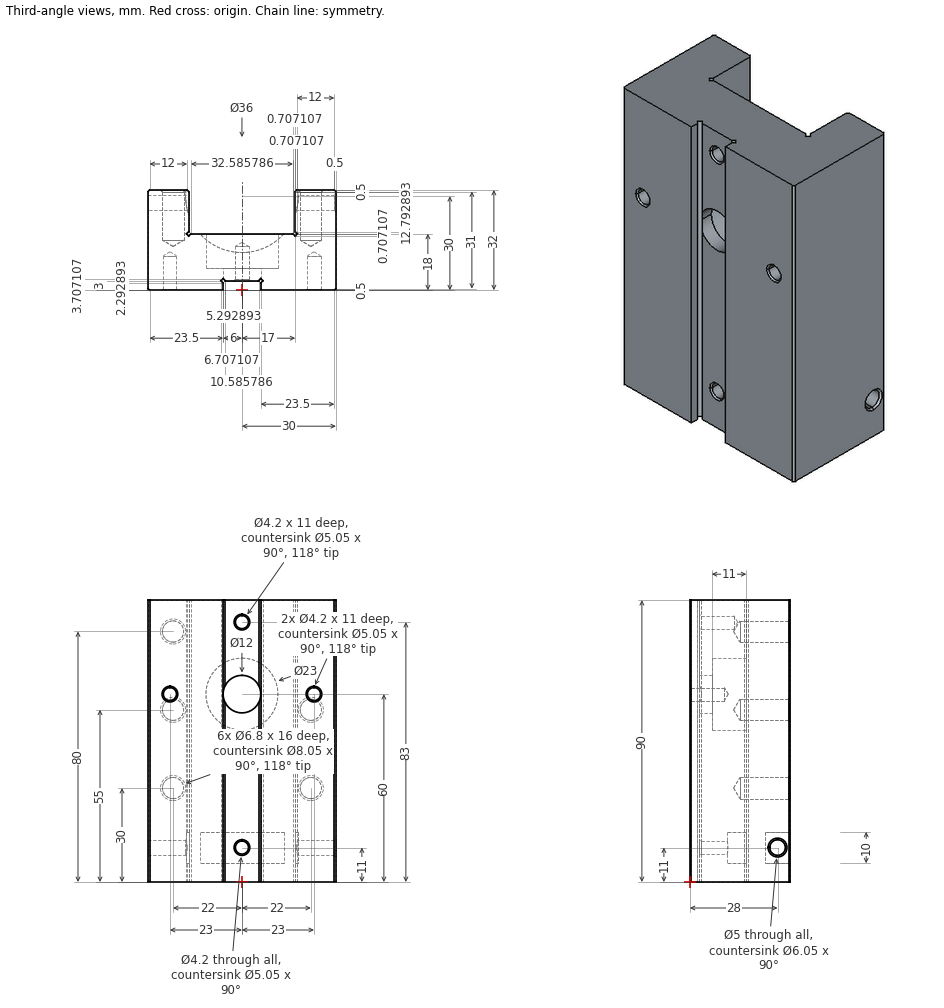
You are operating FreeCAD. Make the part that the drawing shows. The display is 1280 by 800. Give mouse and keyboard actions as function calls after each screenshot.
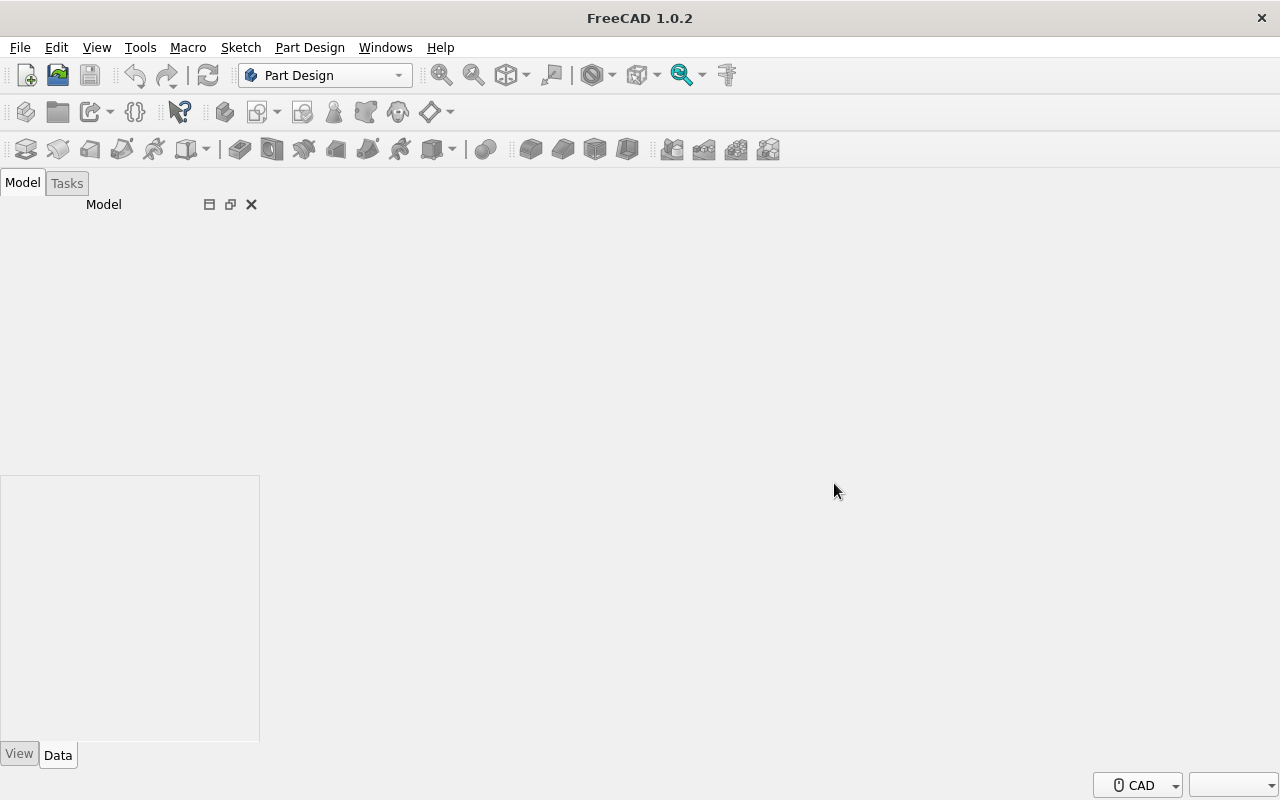
click(26, 76)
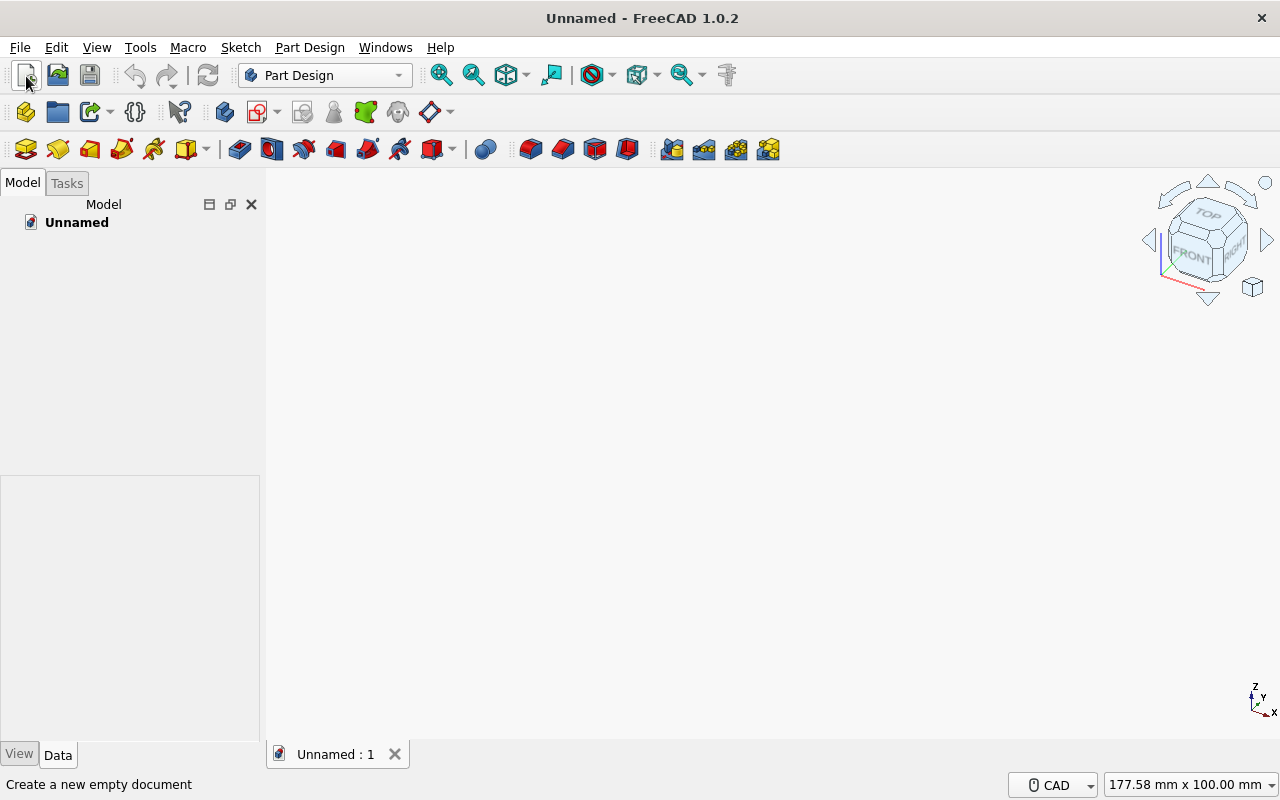
click(258, 112)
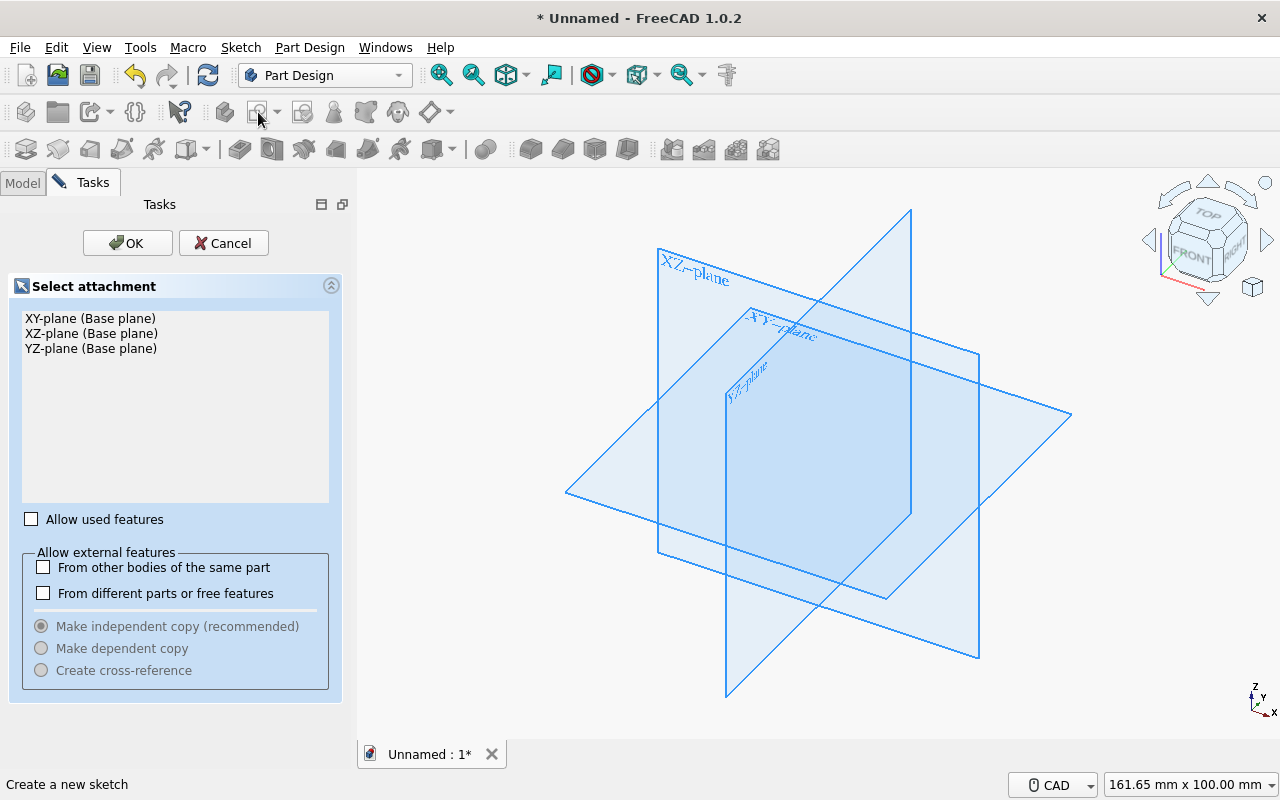
click(82, 318)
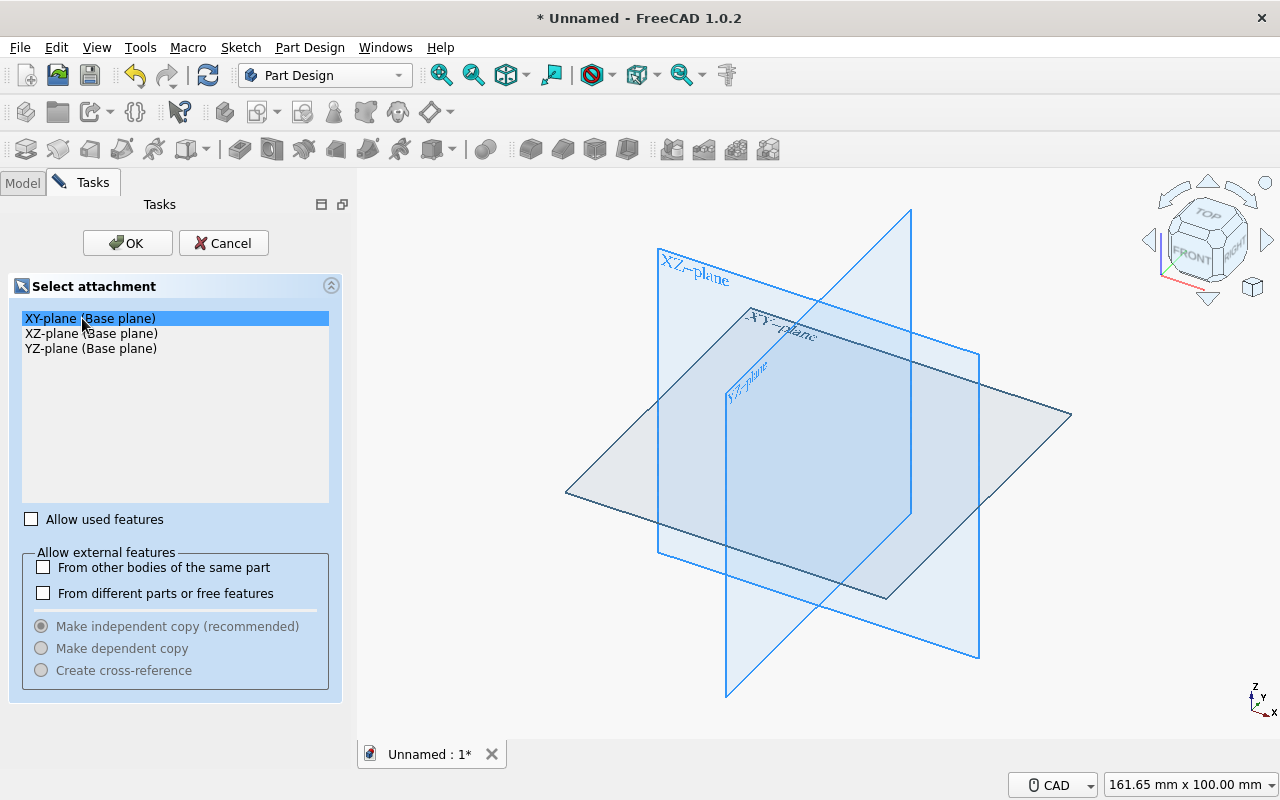
click(128, 243)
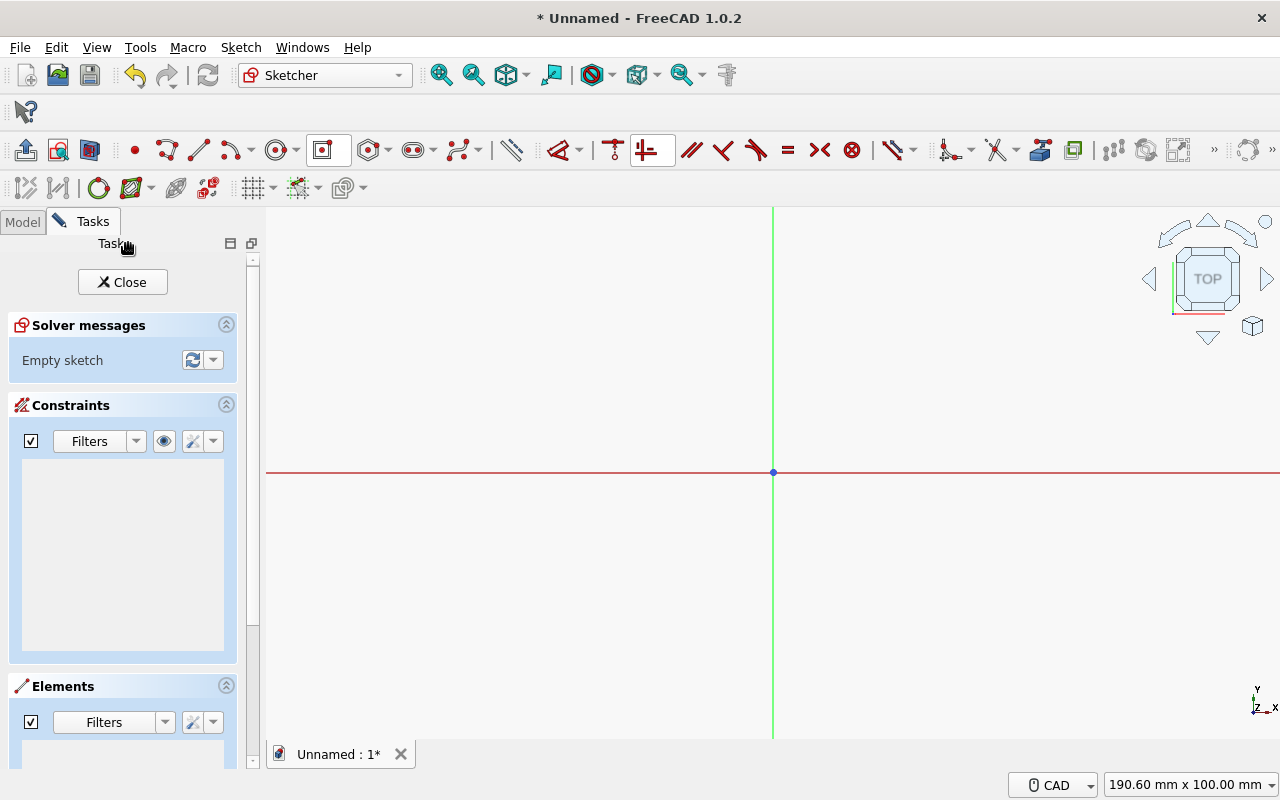
scroll(856, 284, up, 3)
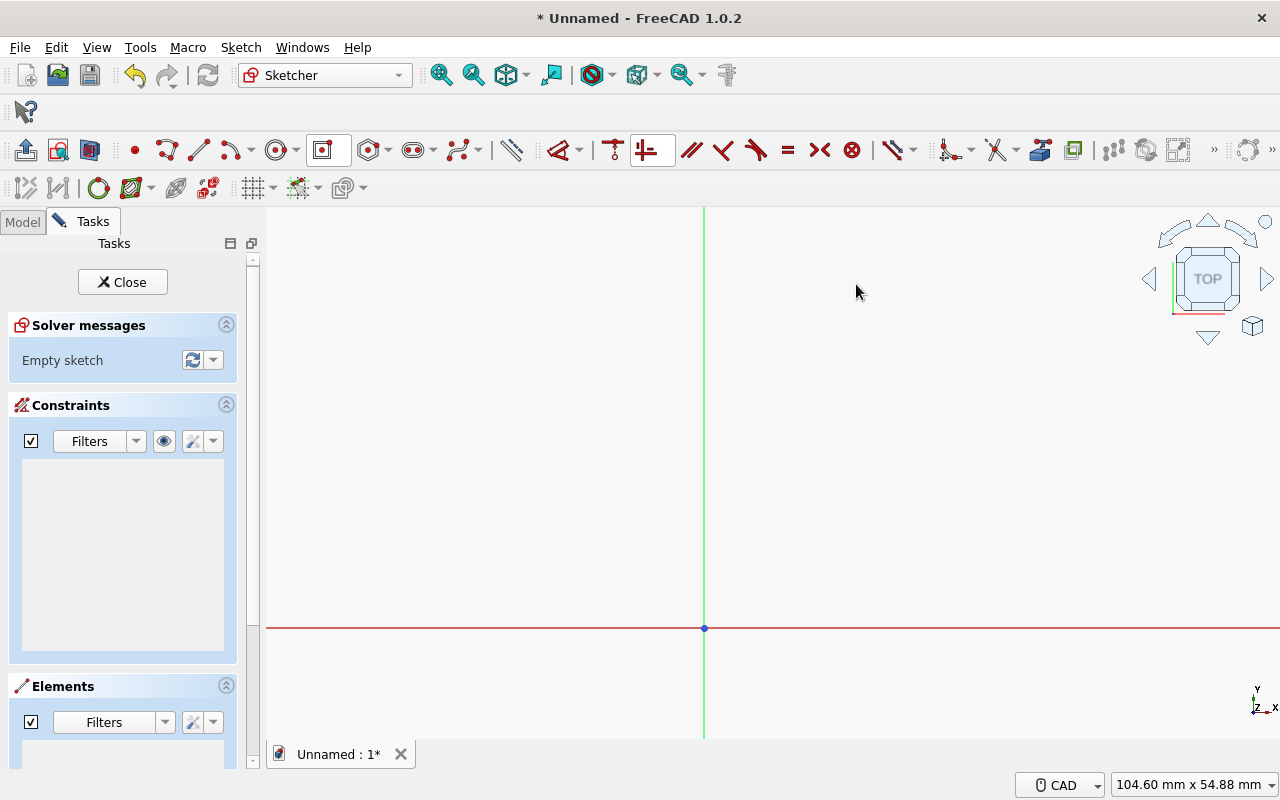
click(168, 150)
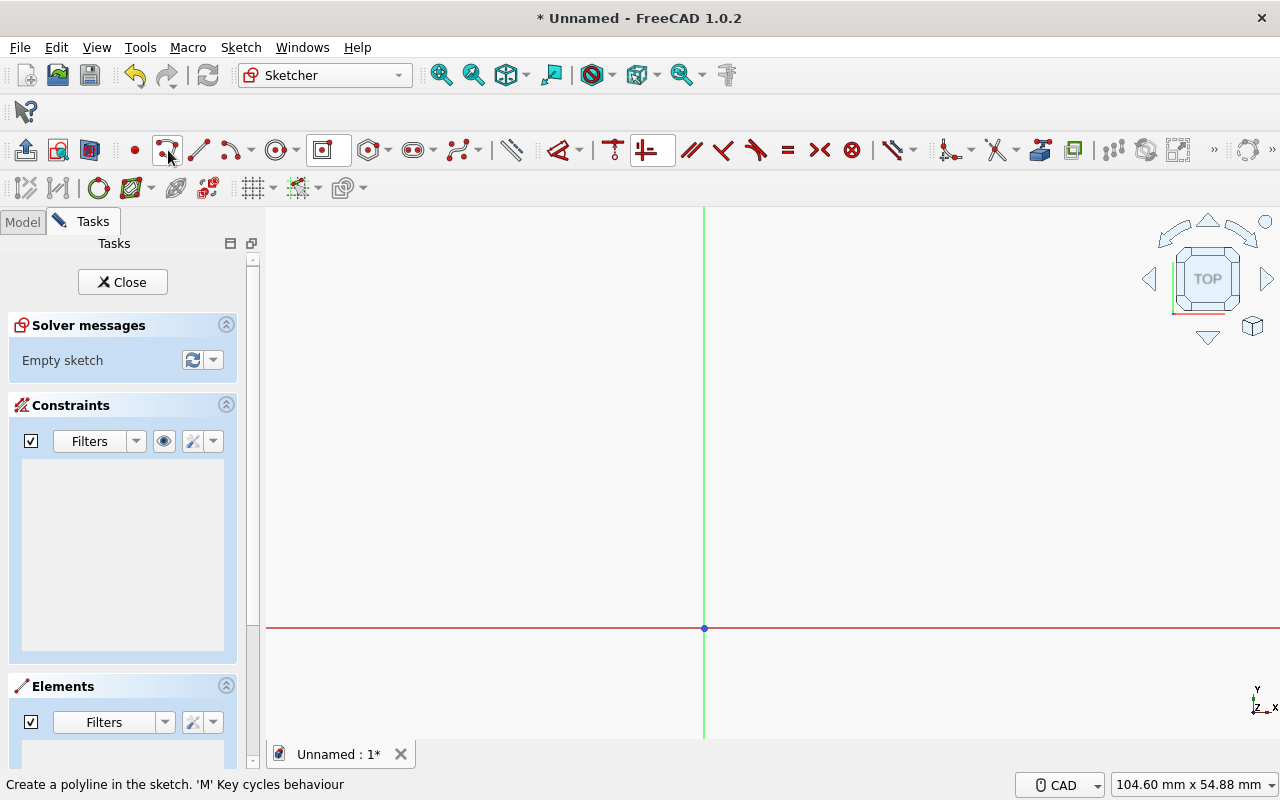
click(646, 628)
click(646, 606)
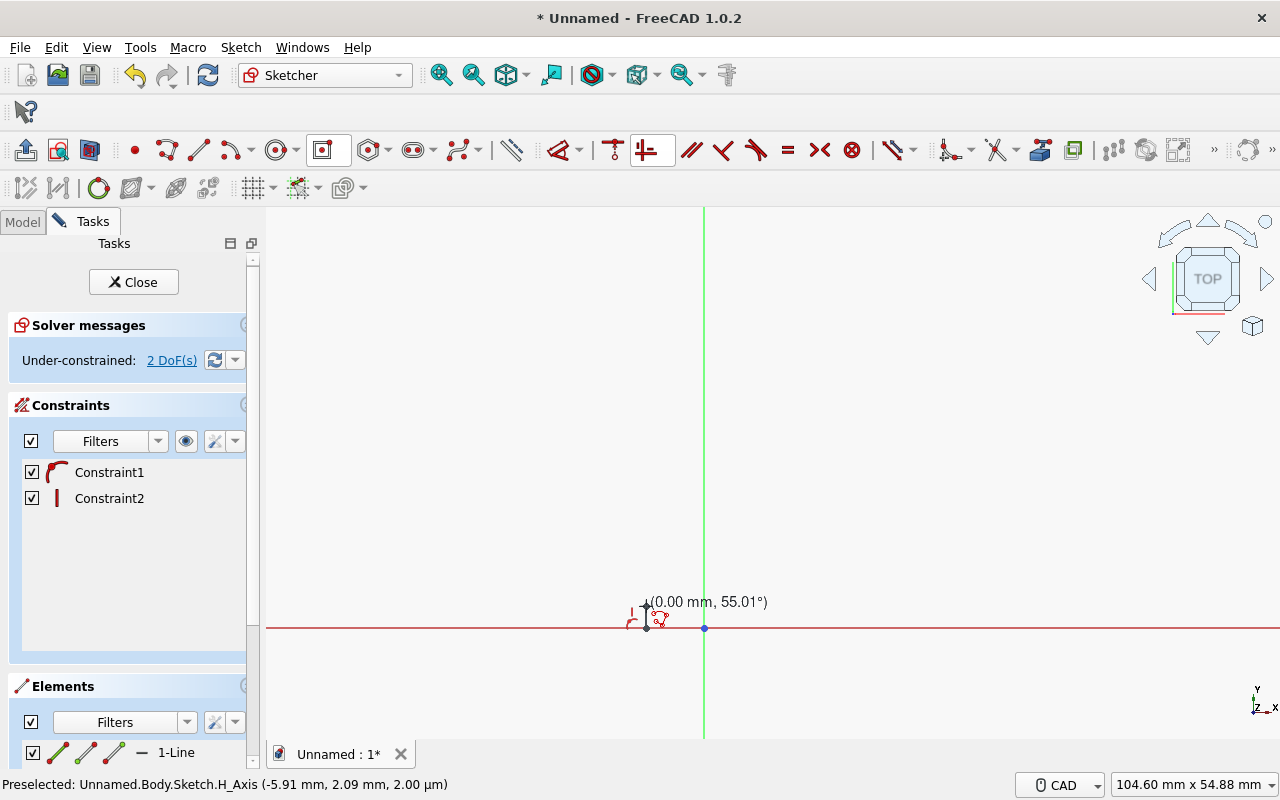
scroll(639, 599, up, 3)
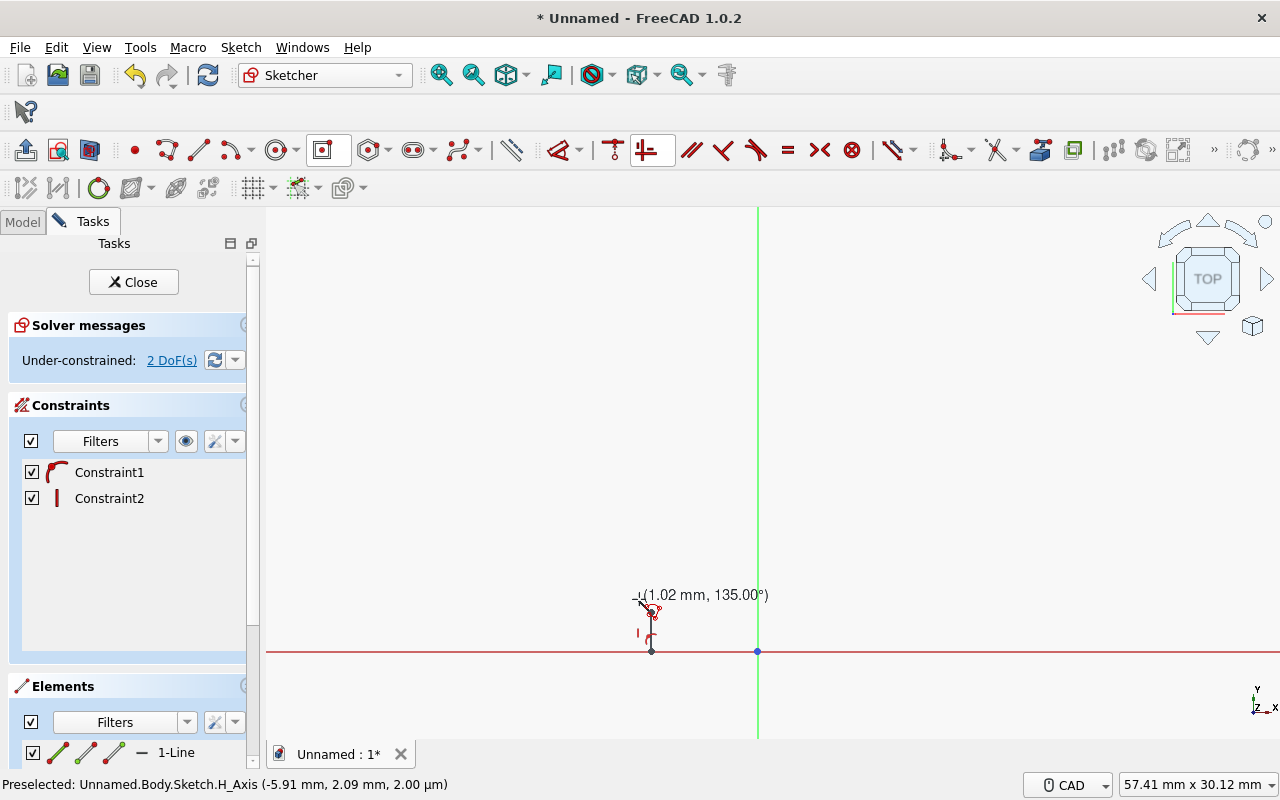
click(639, 599)
click(652, 586)
click(664, 599)
click(851, 599)
click(864, 586)
click(876, 599)
click(864, 611)
click(864, 652)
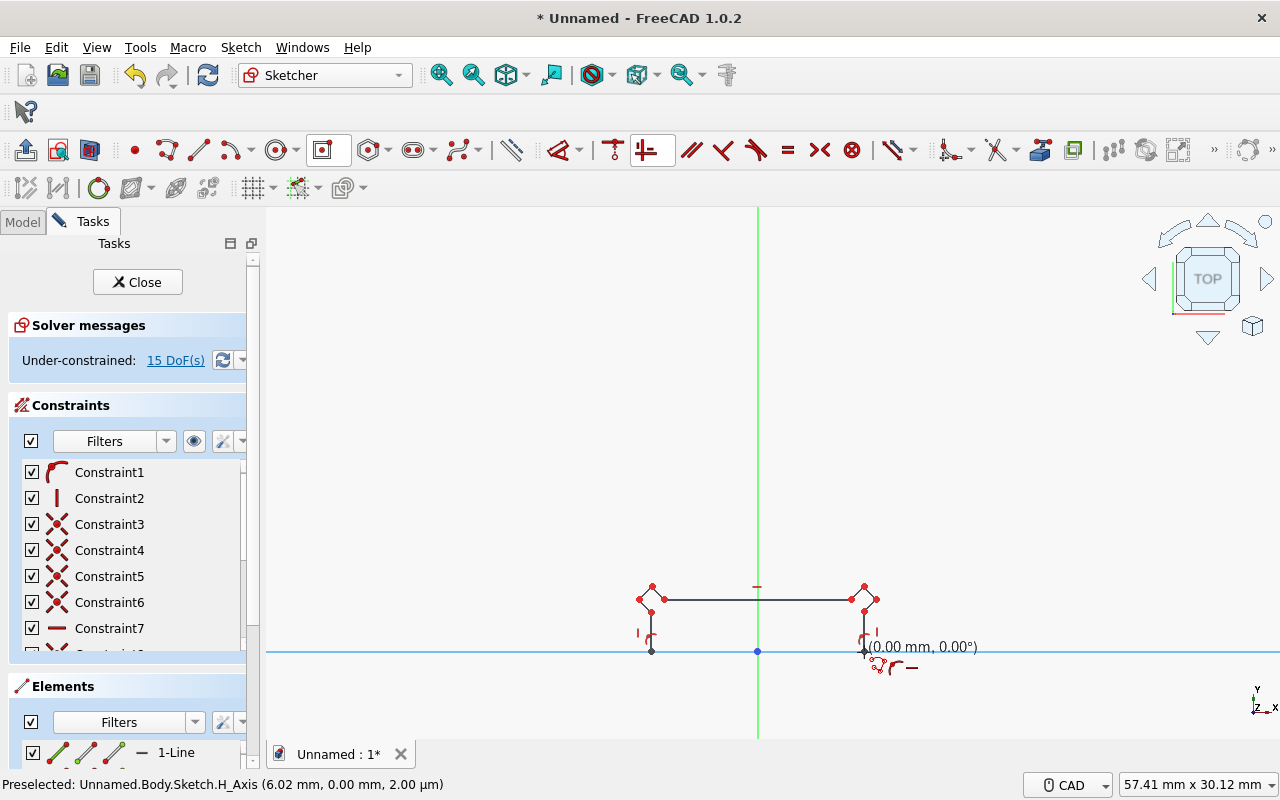
scroll(640, 599, down, 3)